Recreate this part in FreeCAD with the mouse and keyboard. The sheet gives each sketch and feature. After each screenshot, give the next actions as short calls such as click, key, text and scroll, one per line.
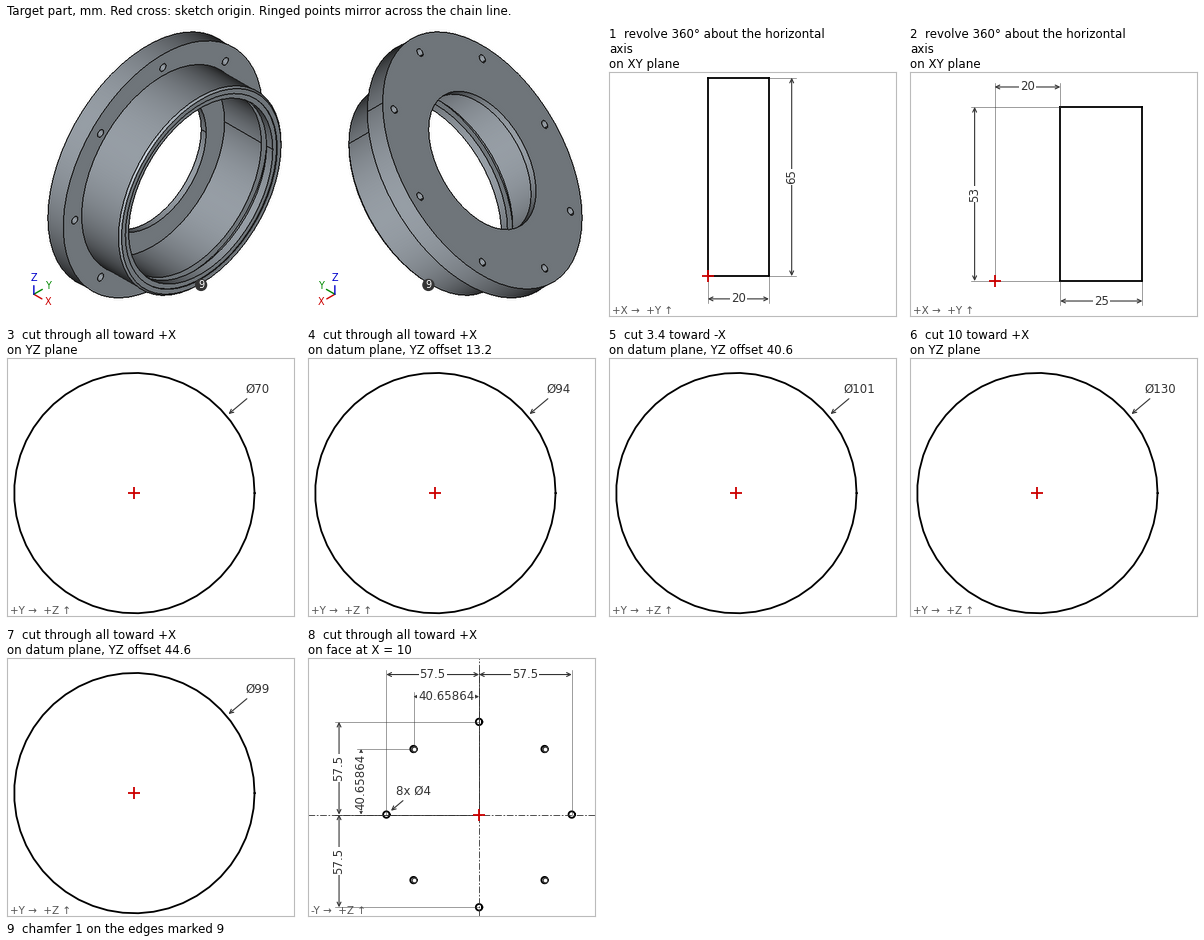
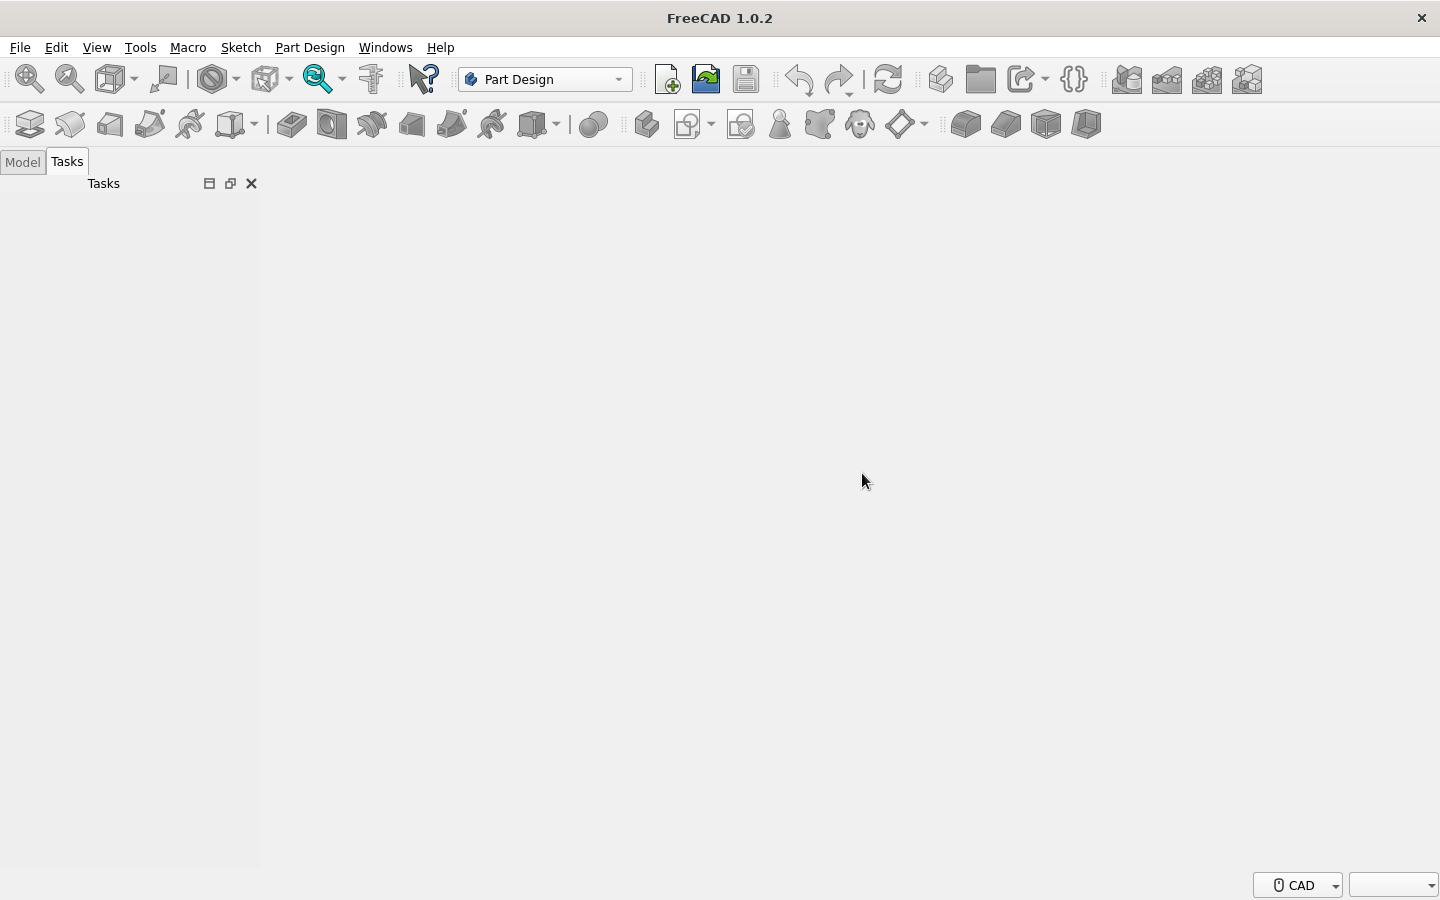
click(666, 80)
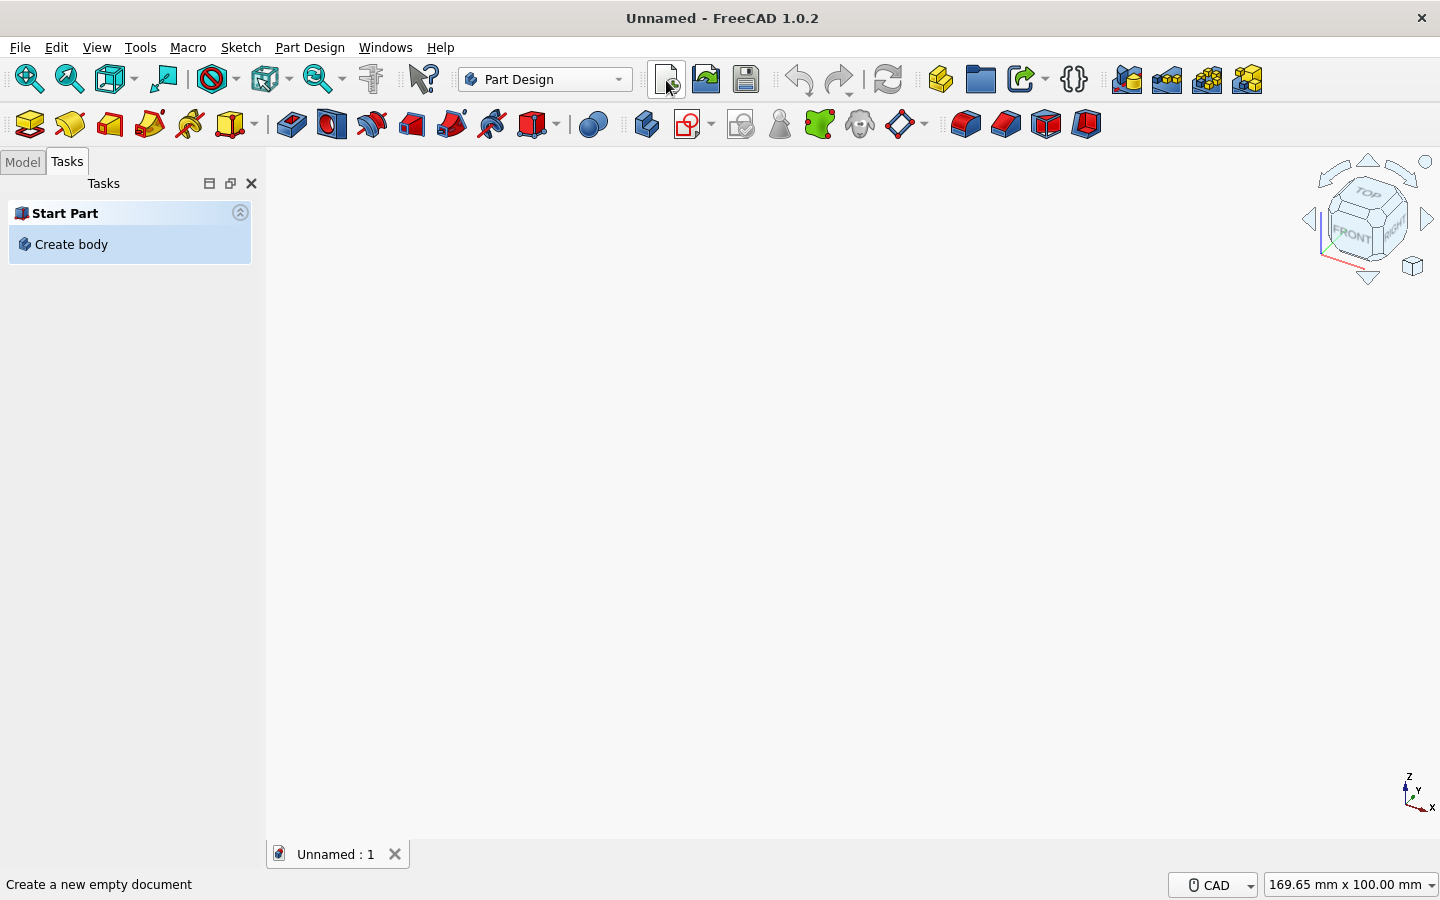
click(688, 124)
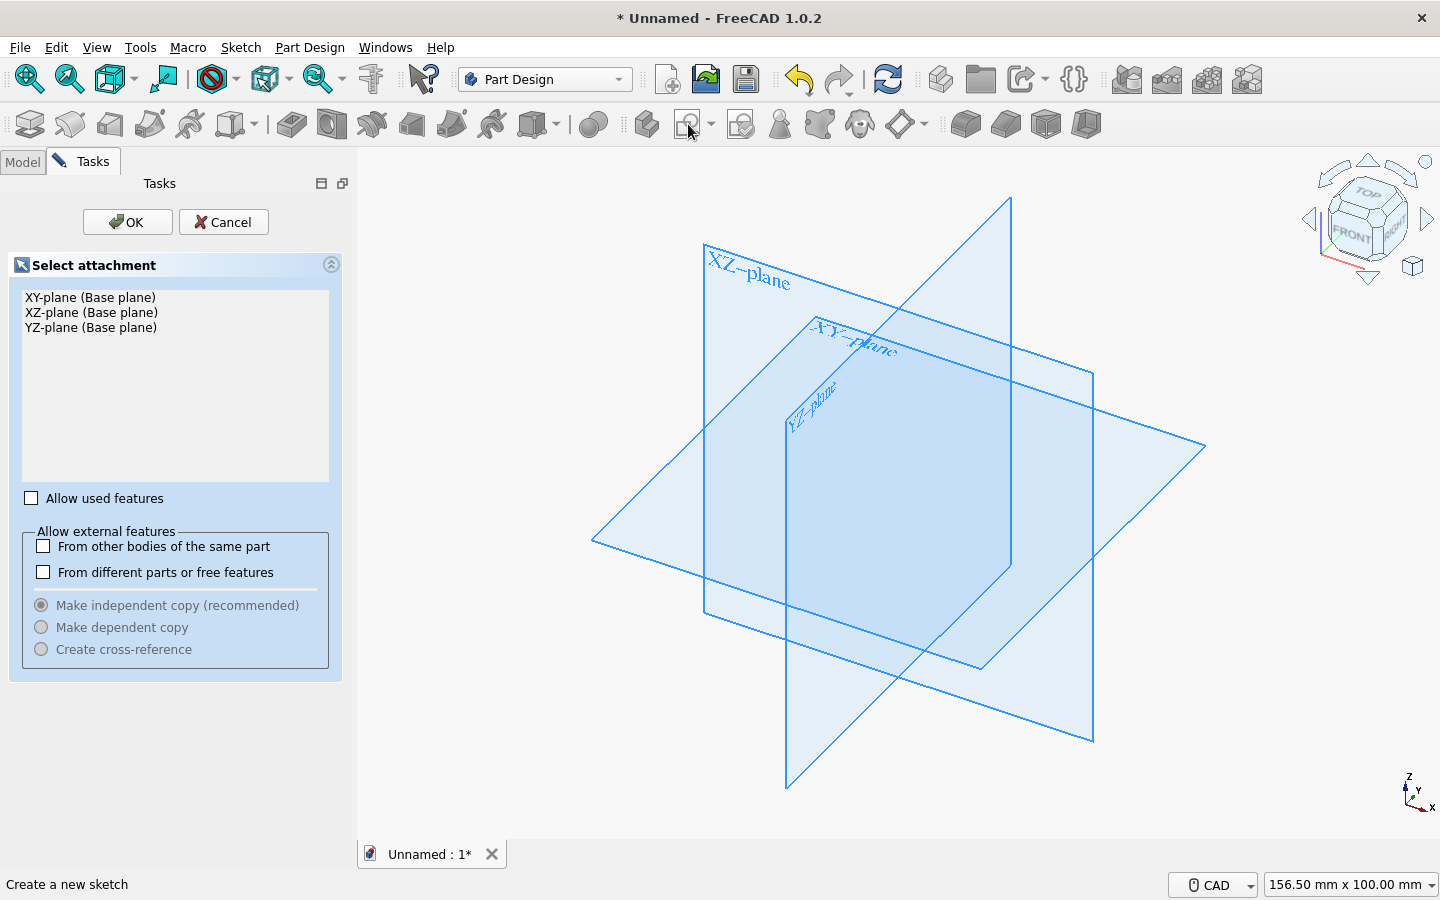
click(82, 298)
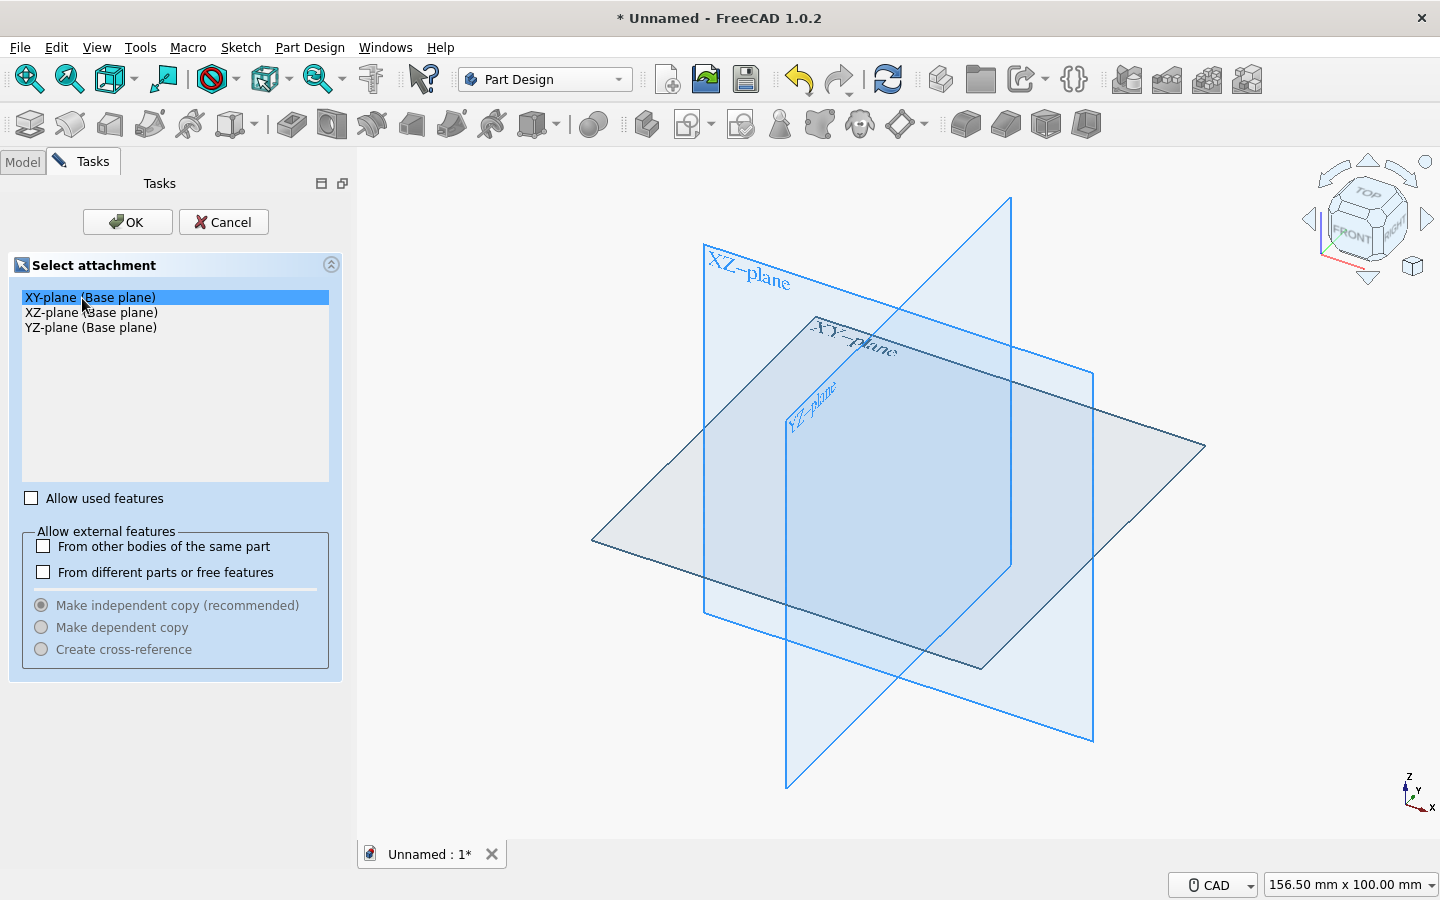
click(128, 222)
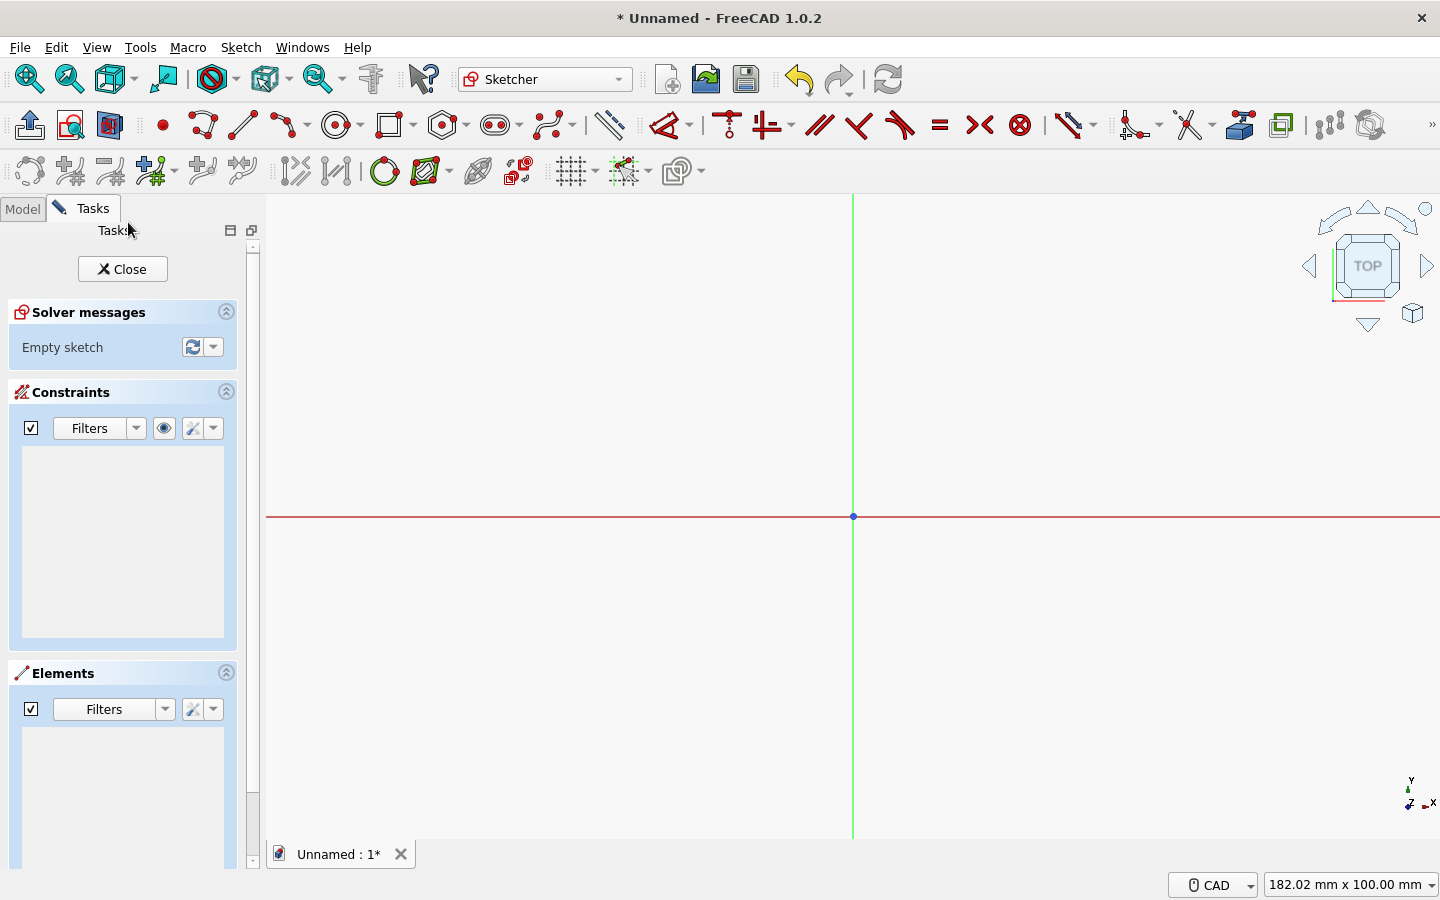
scroll(514, 811, down, 2)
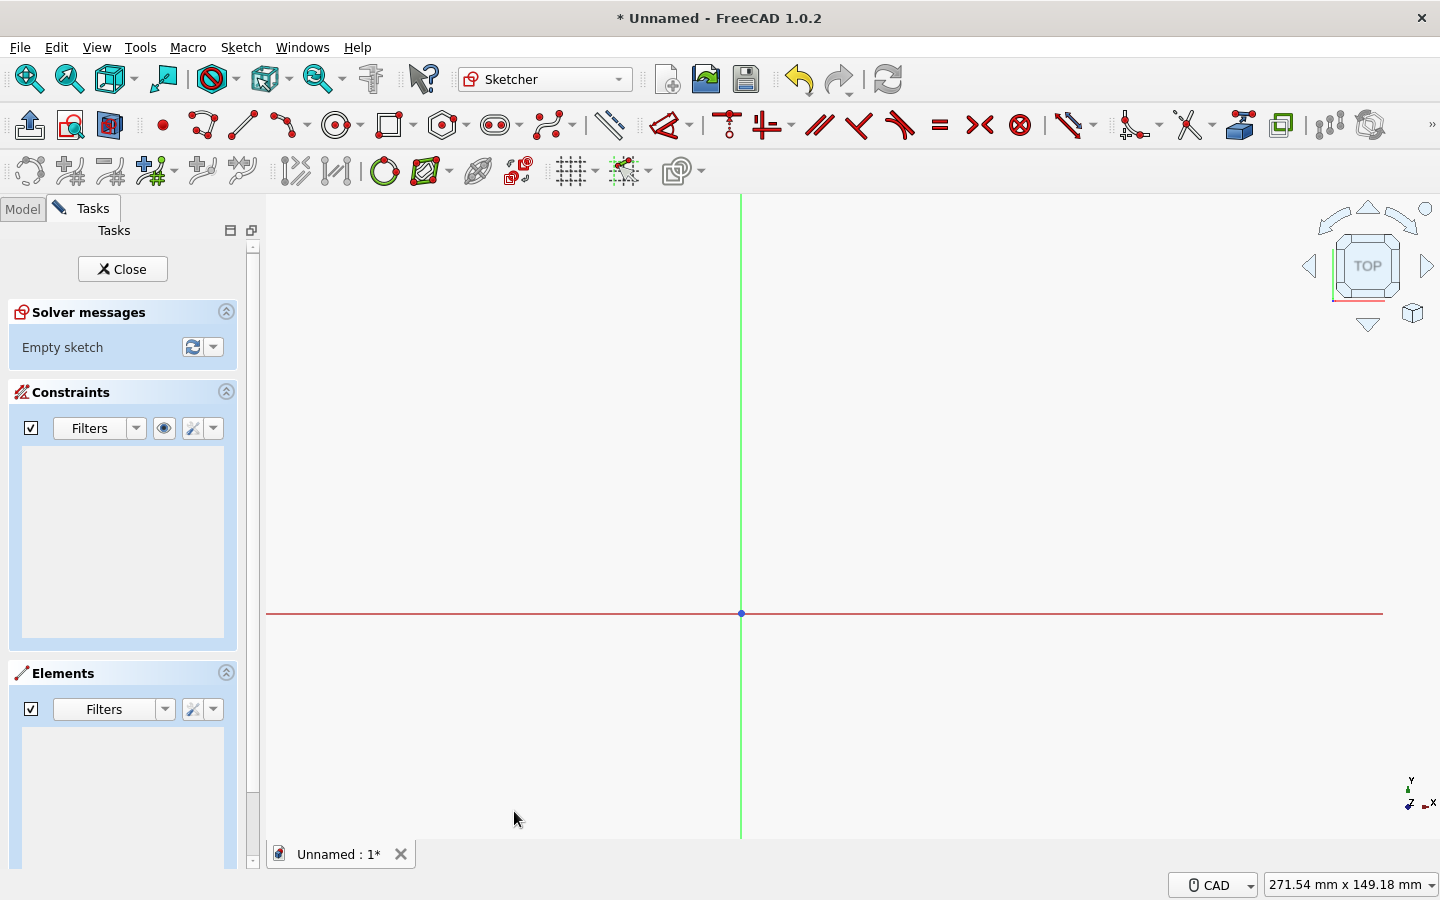
scroll(785, 386, up, 2)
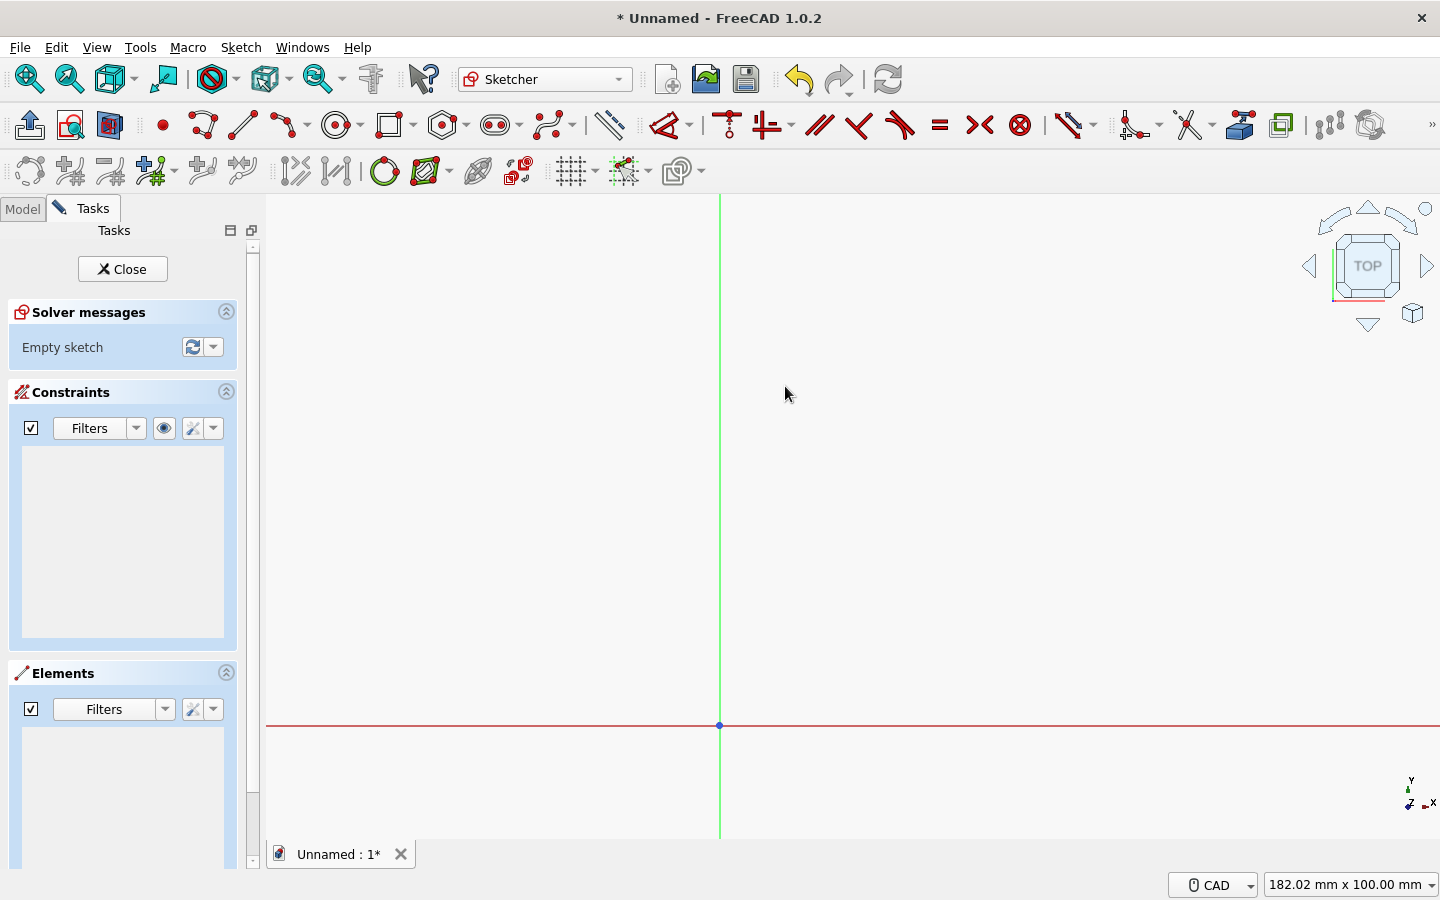
click(390, 126)